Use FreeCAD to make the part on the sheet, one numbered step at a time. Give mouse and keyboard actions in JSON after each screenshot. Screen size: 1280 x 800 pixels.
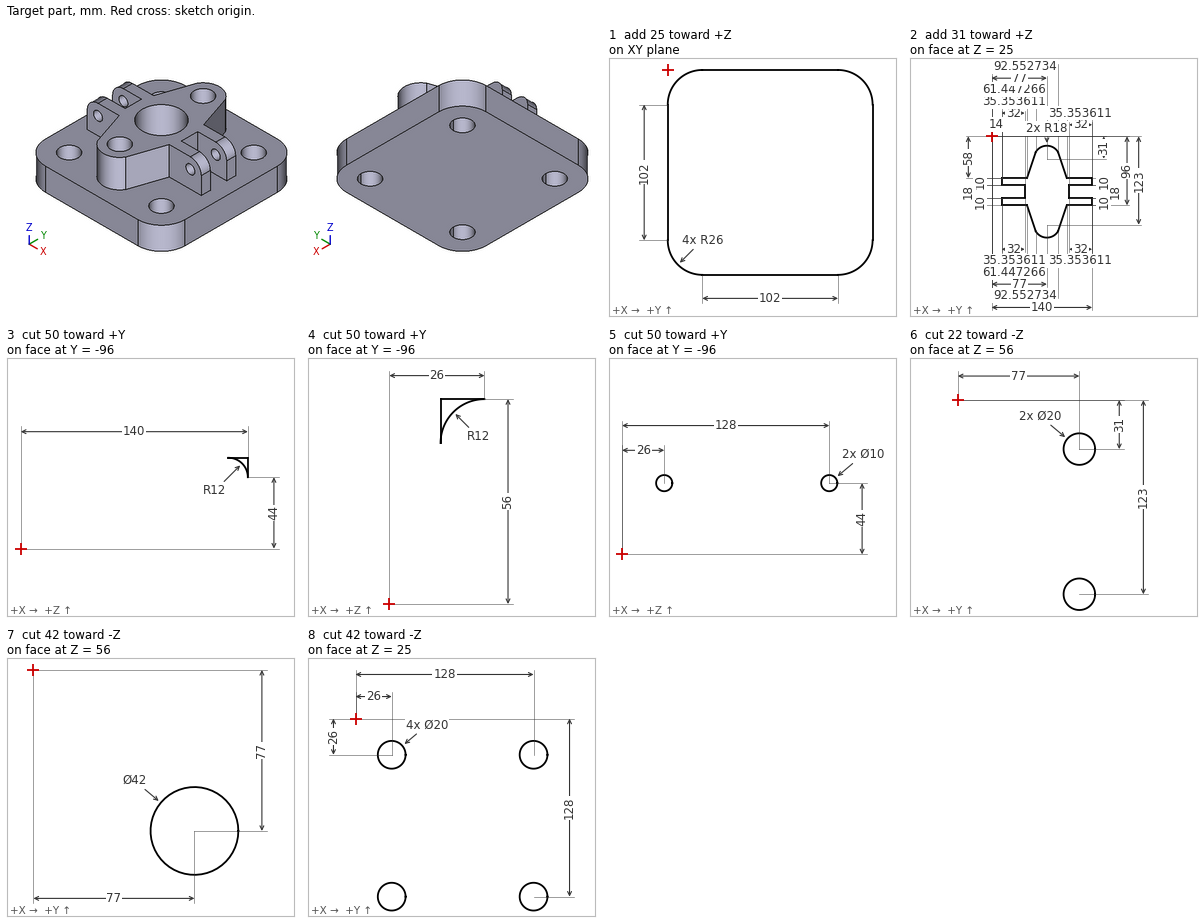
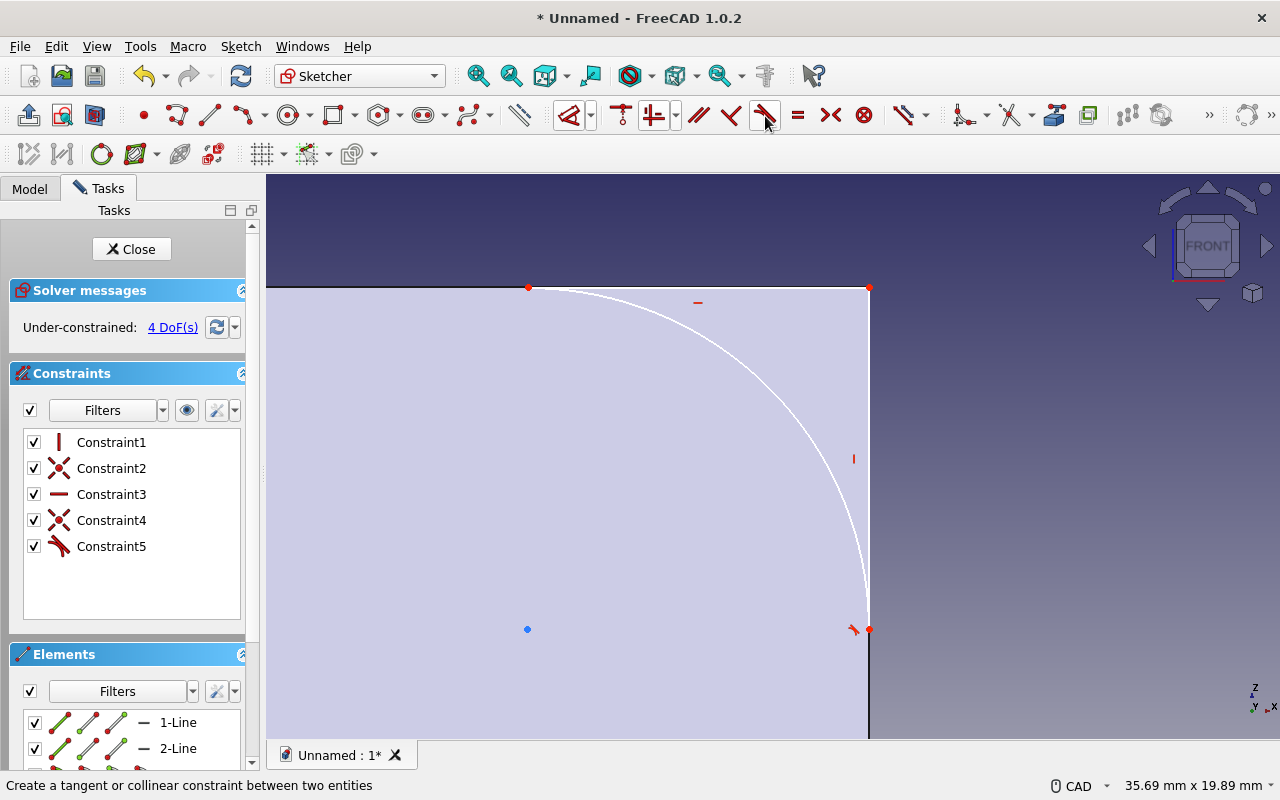
{"action": "left_click", "coordinate": [767, 288]}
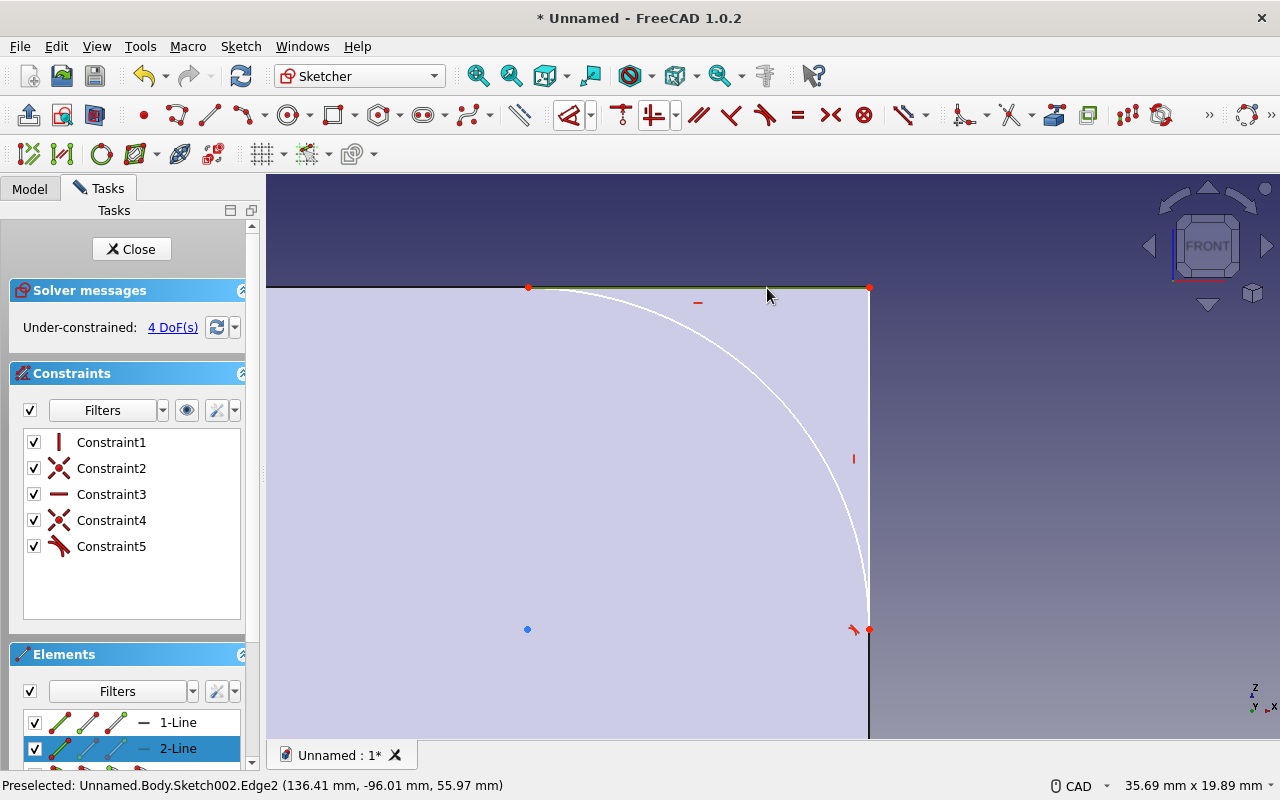
{"action": "left_click", "coordinate": [832, 475]}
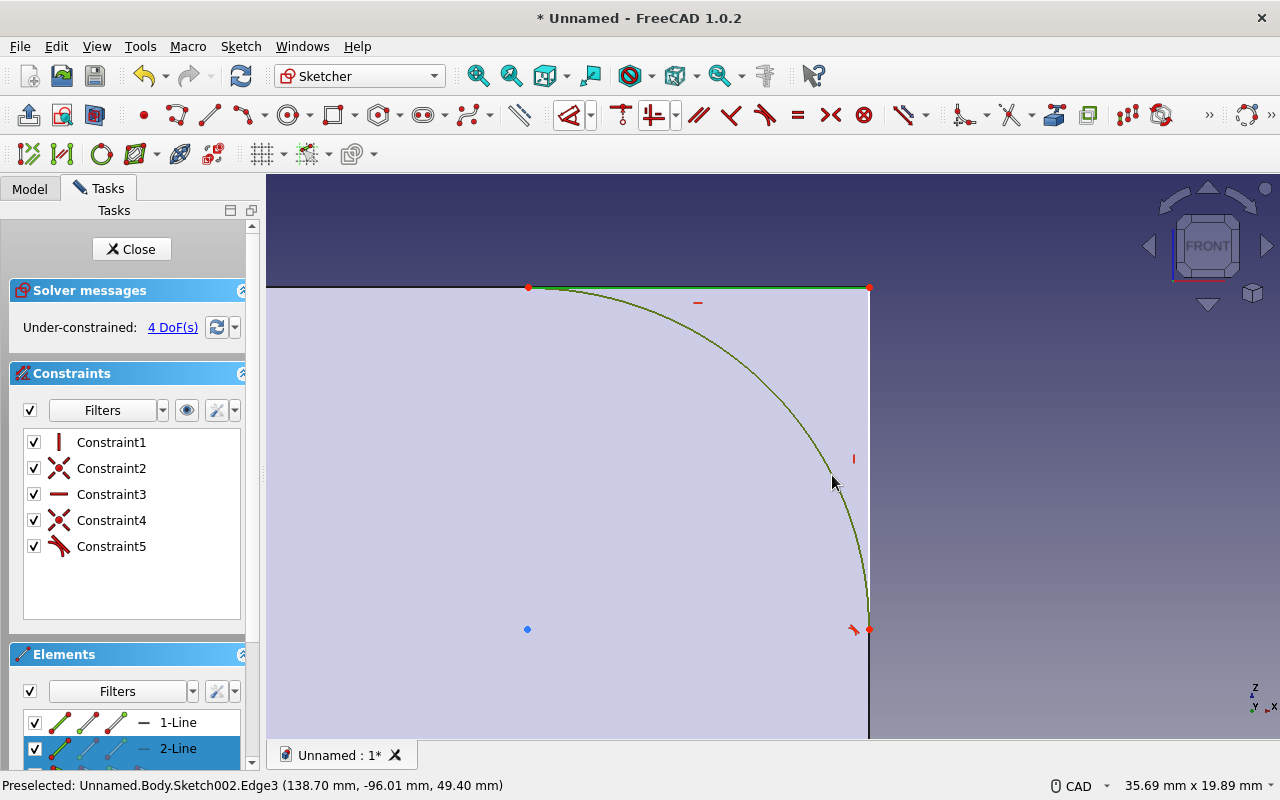
{"action": "left_click", "coordinate": [765, 116]}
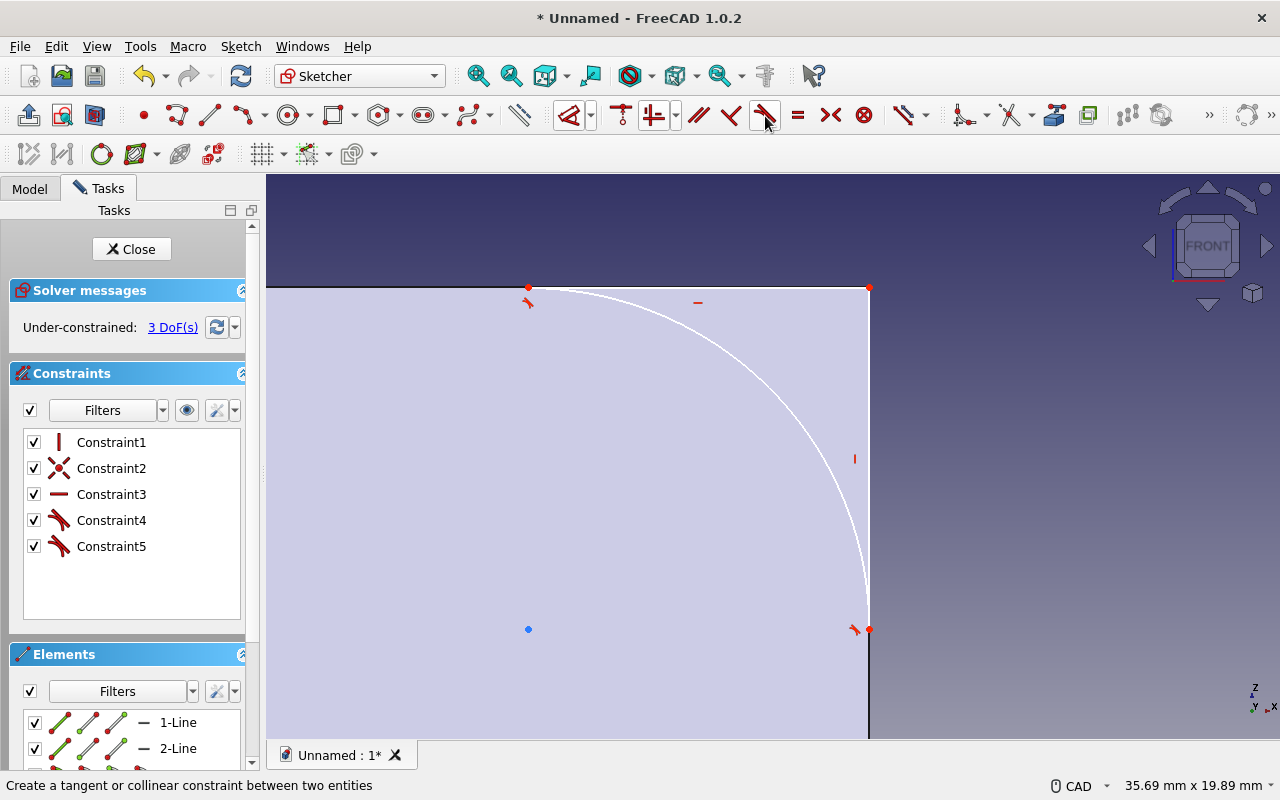
{"action": "left_click", "coordinate": [832, 474]}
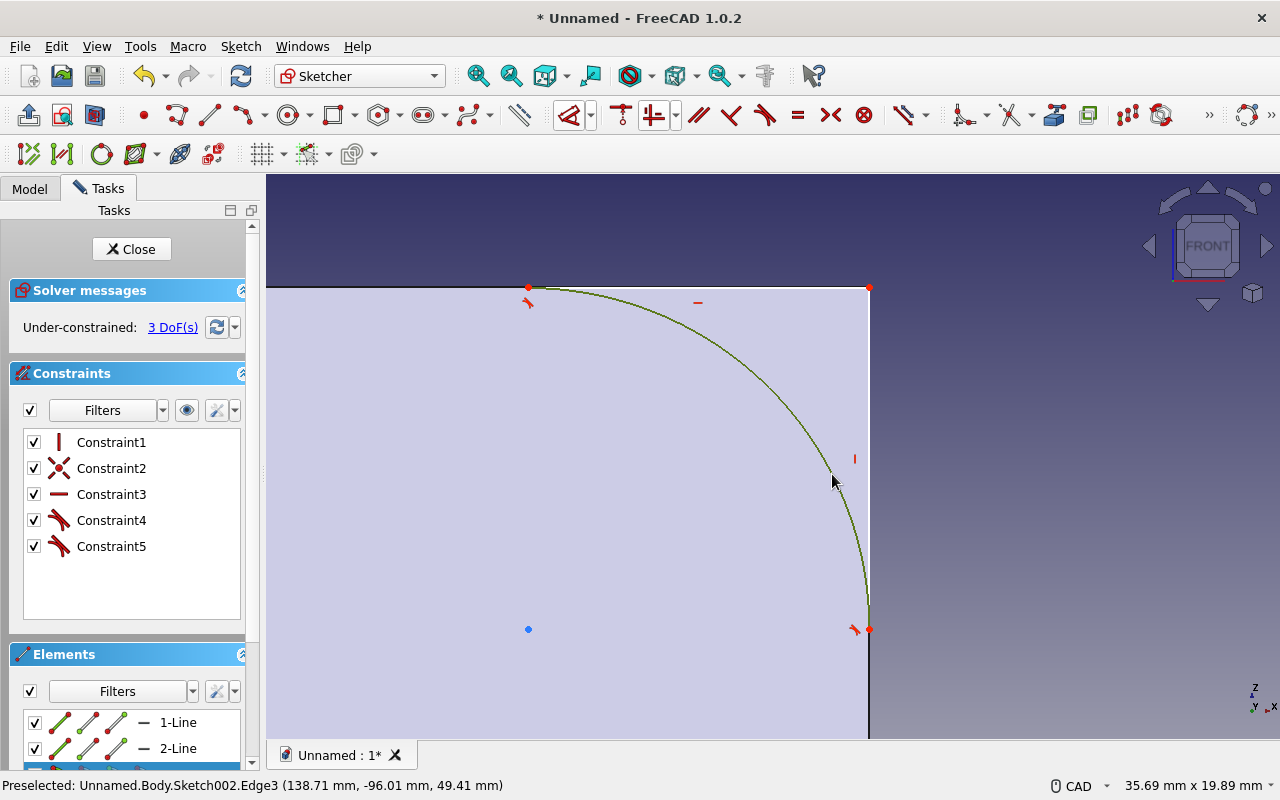
{"action": "key", "text": "k r"}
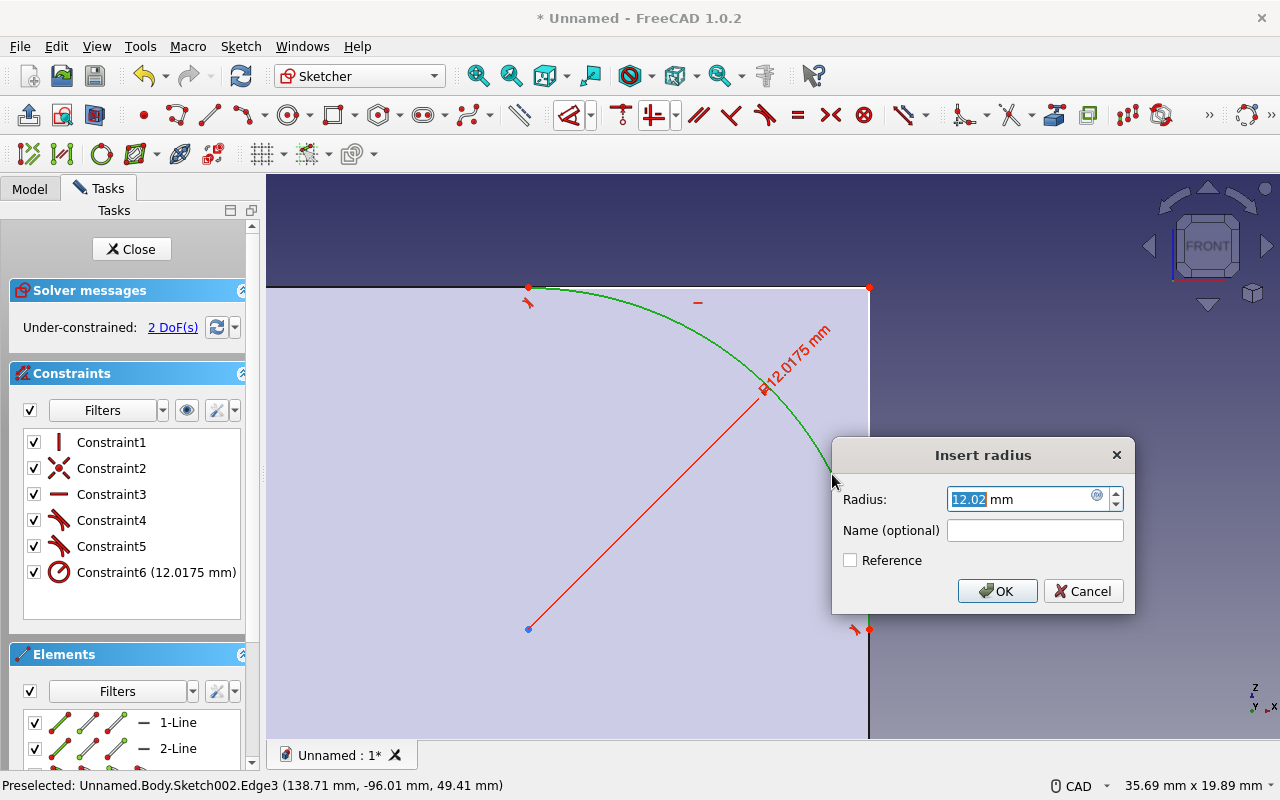
{"action": "type", "text": "12"}
{"action": "key", "text": "Return"}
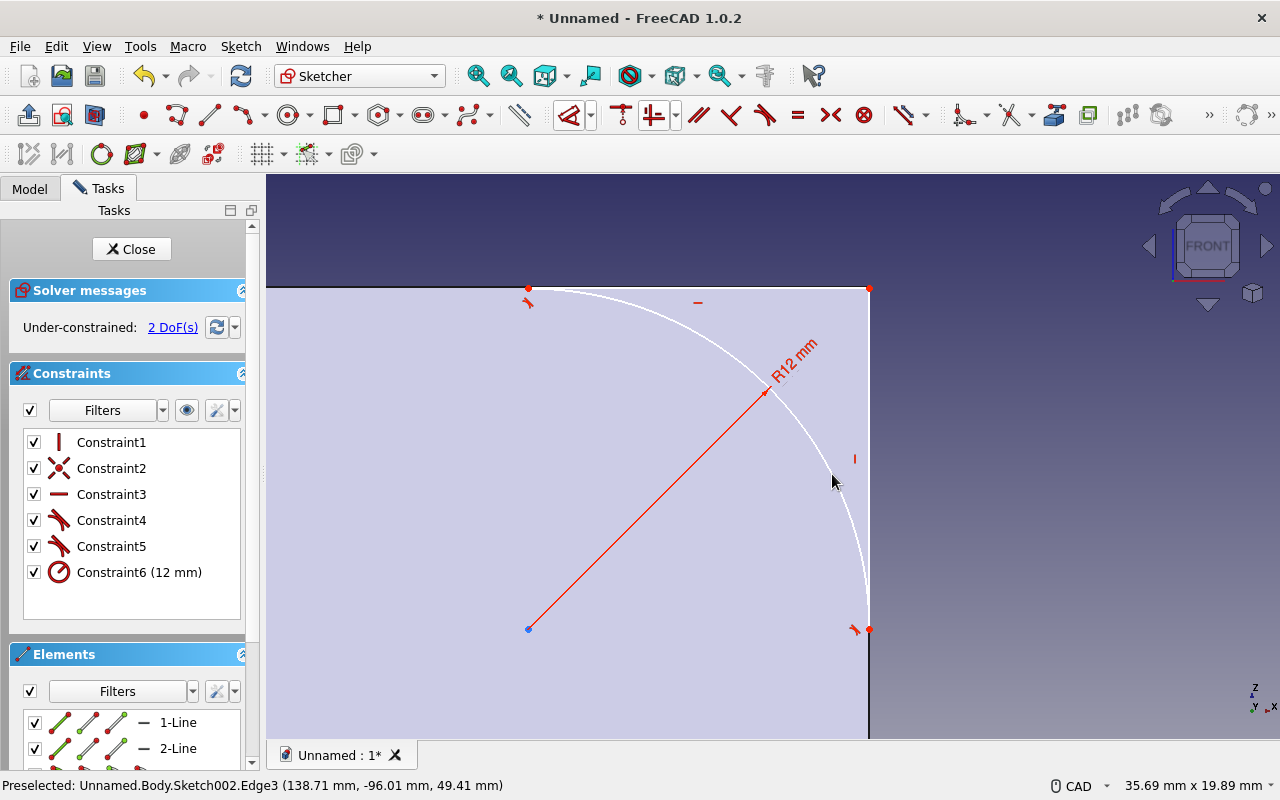
{"action": "left_click", "coordinate": [869, 629]}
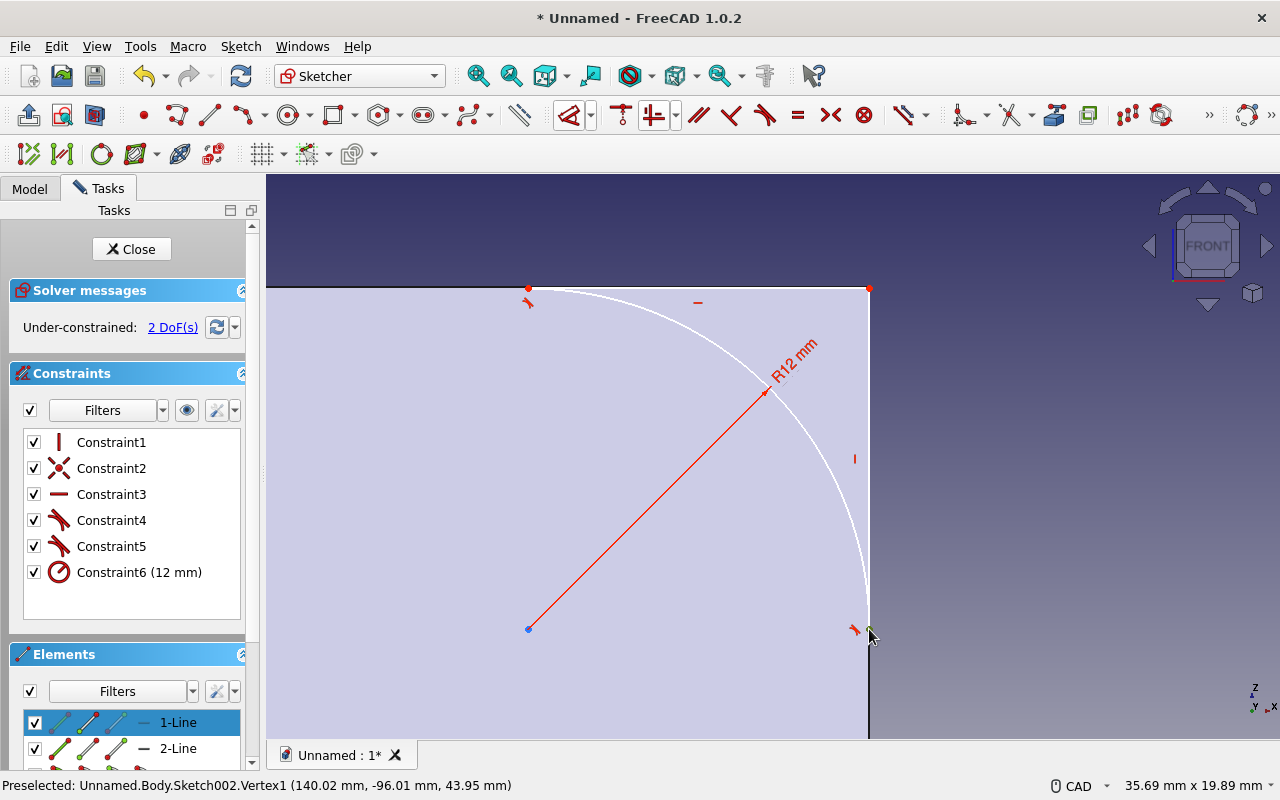
{"action": "left_click", "coordinate": [590, 116]}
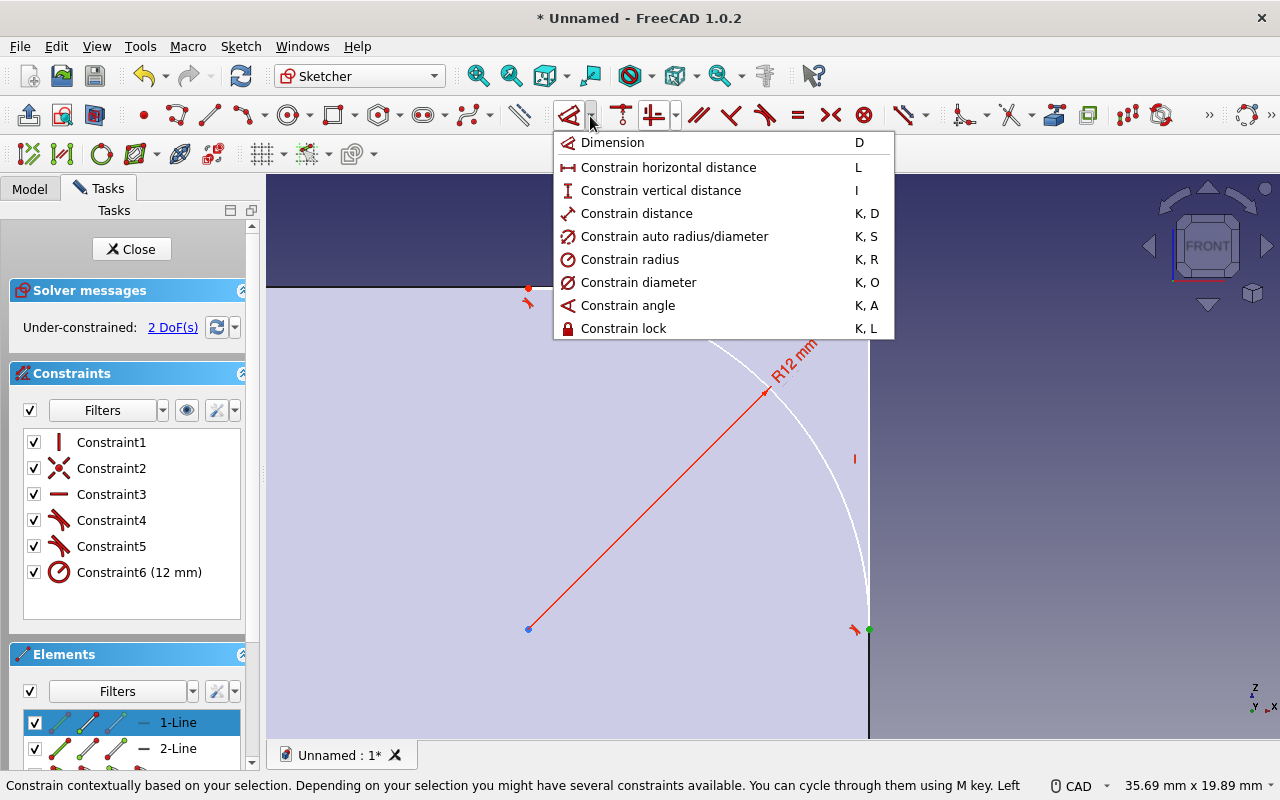
{"action": "left_click", "coordinate": [724, 190]}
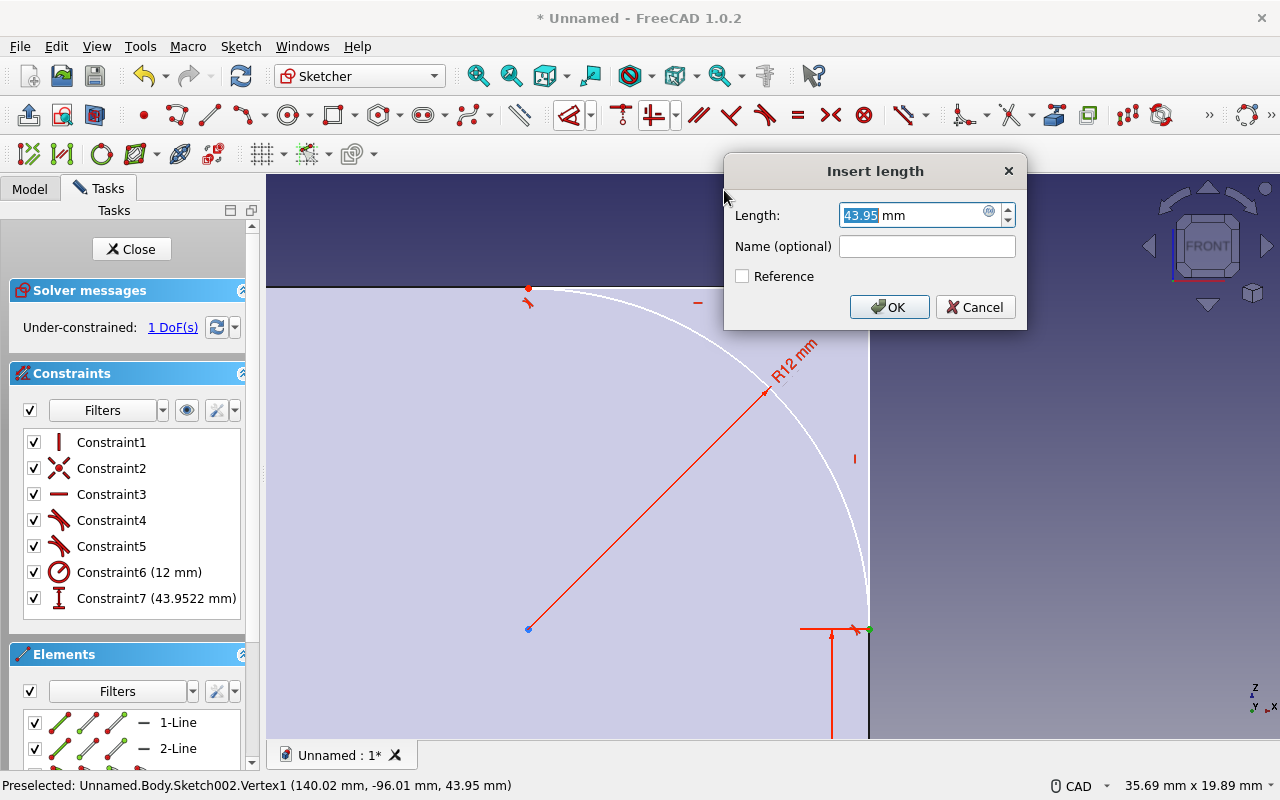
{"action": "type", "text": "44"}
{"action": "key", "text": "Return"}